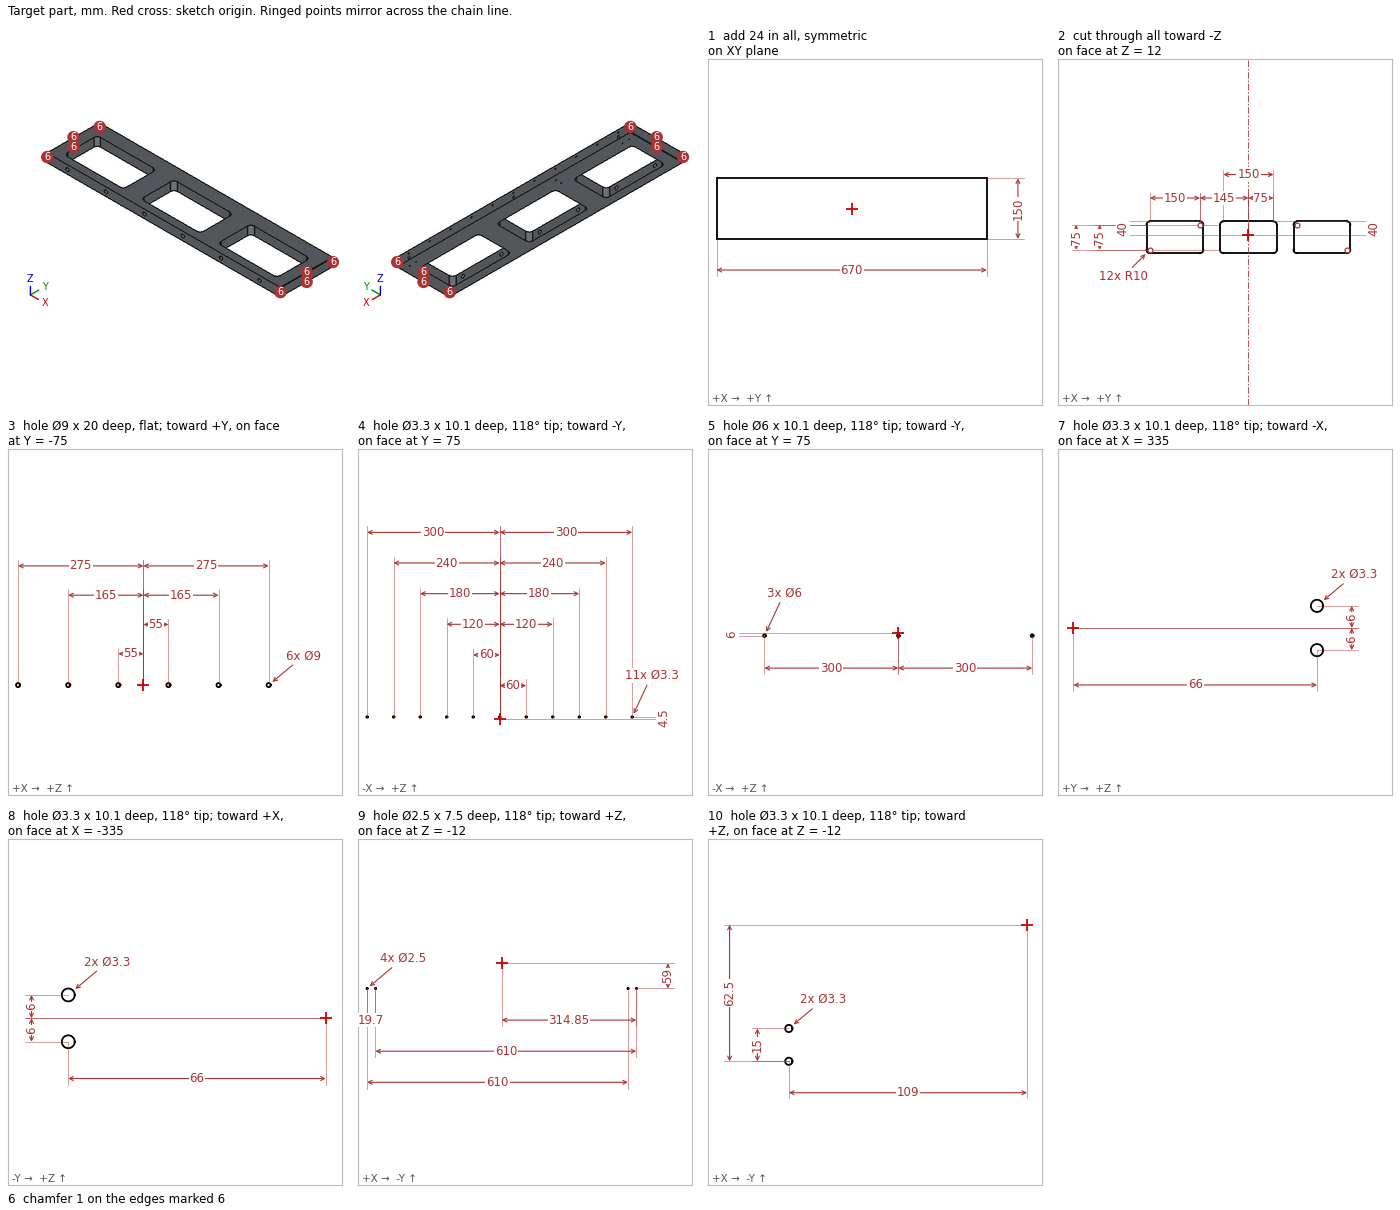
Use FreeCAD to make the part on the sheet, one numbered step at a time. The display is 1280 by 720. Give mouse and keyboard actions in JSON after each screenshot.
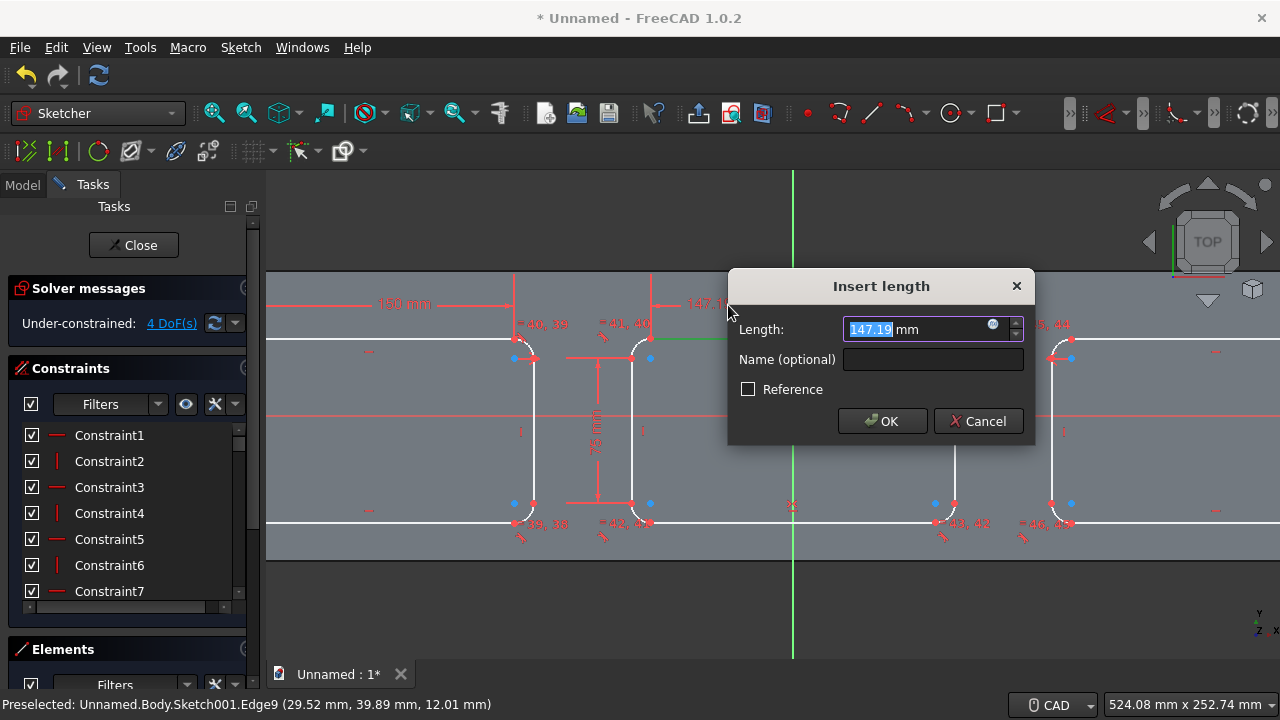
{"action": "type", "text": "150"}
{"action": "key", "text": "Return"}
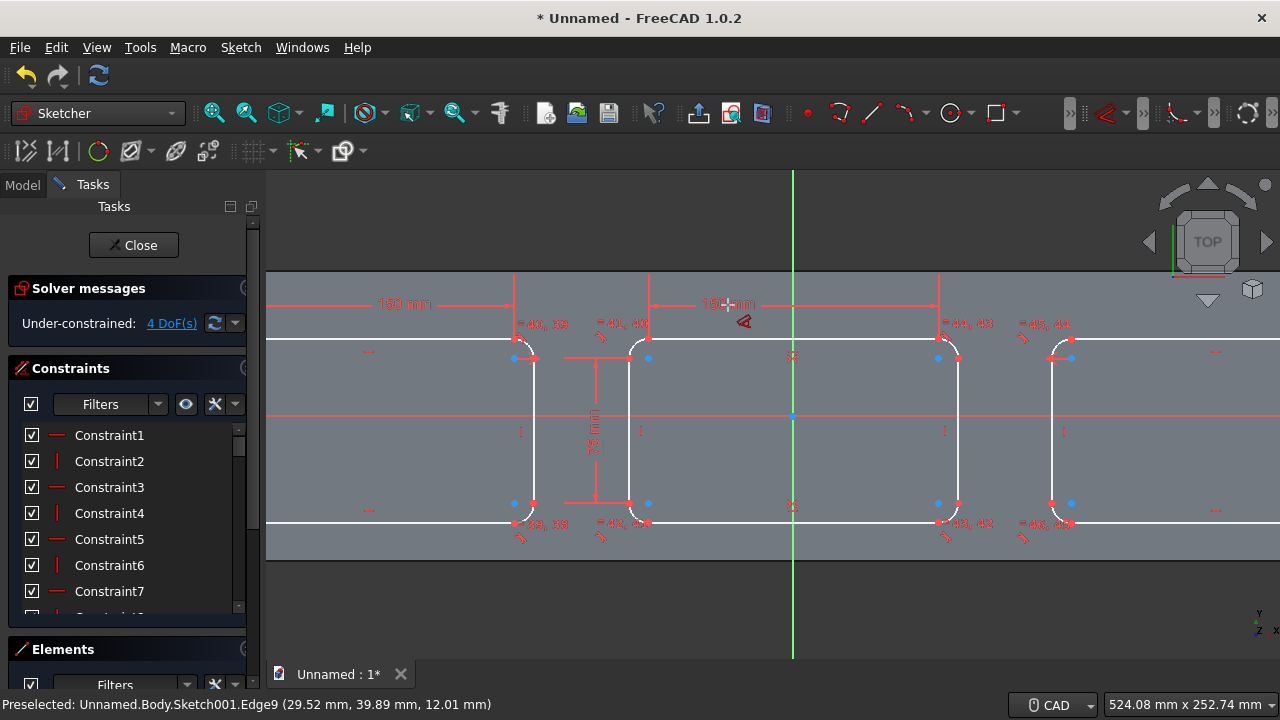
{"action": "left_click", "coordinate": [514, 339]}
{"action": "left_click", "coordinate": [480, 378]}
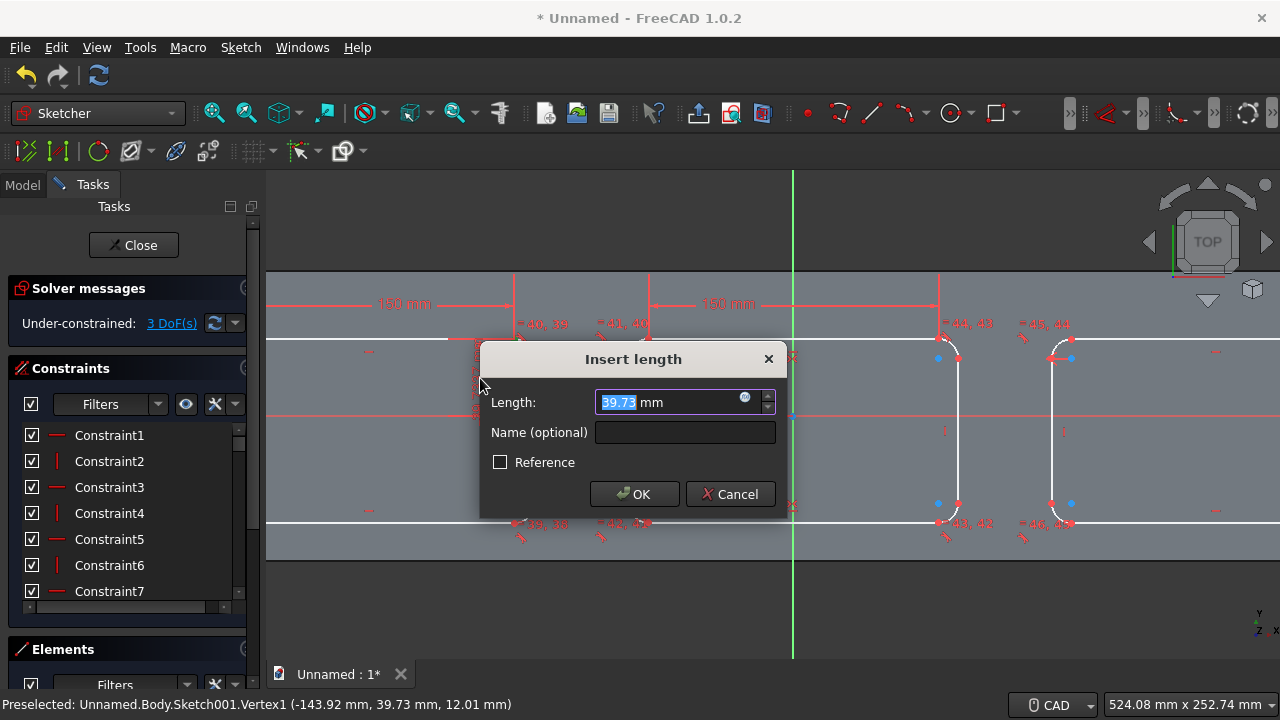
{"action": "type", "text": "40"}
{"action": "key", "text": "Return"}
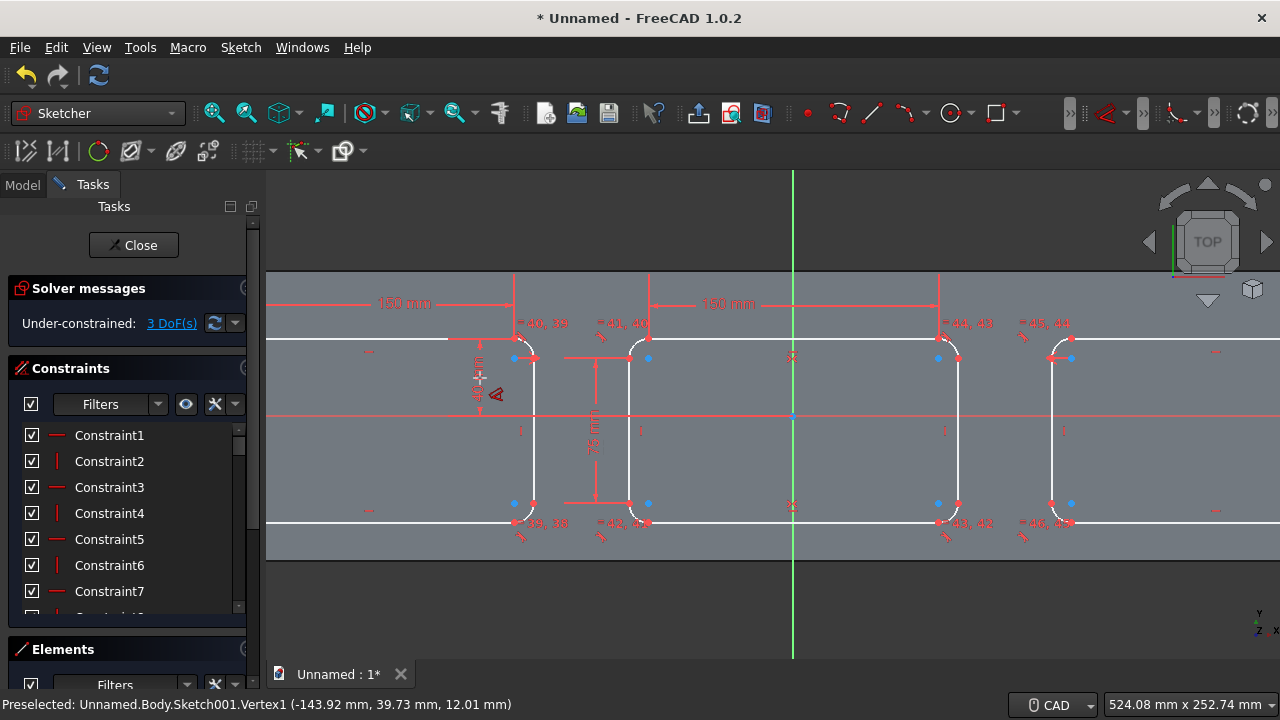
{"action": "left_click", "coordinate": [939, 339]}
{"action": "left_click", "coordinate": [866, 305]}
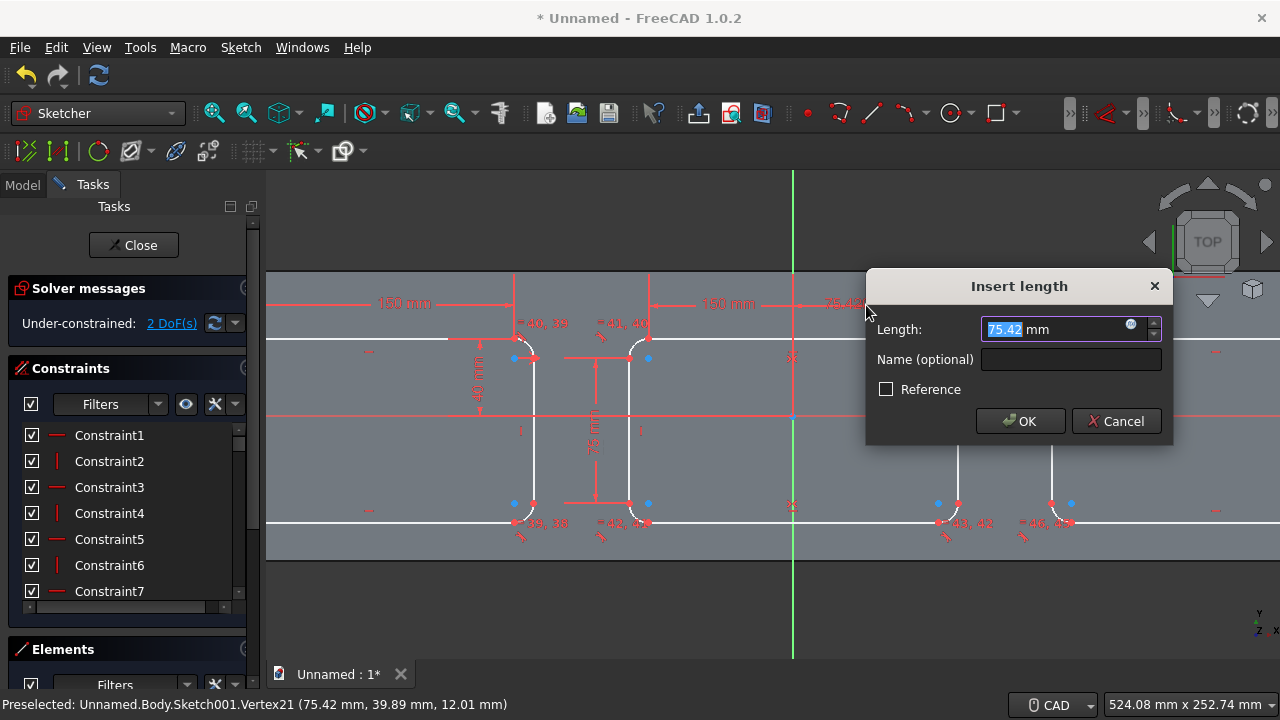
{"action": "type", "text": "75"}
{"action": "key", "text": "Return"}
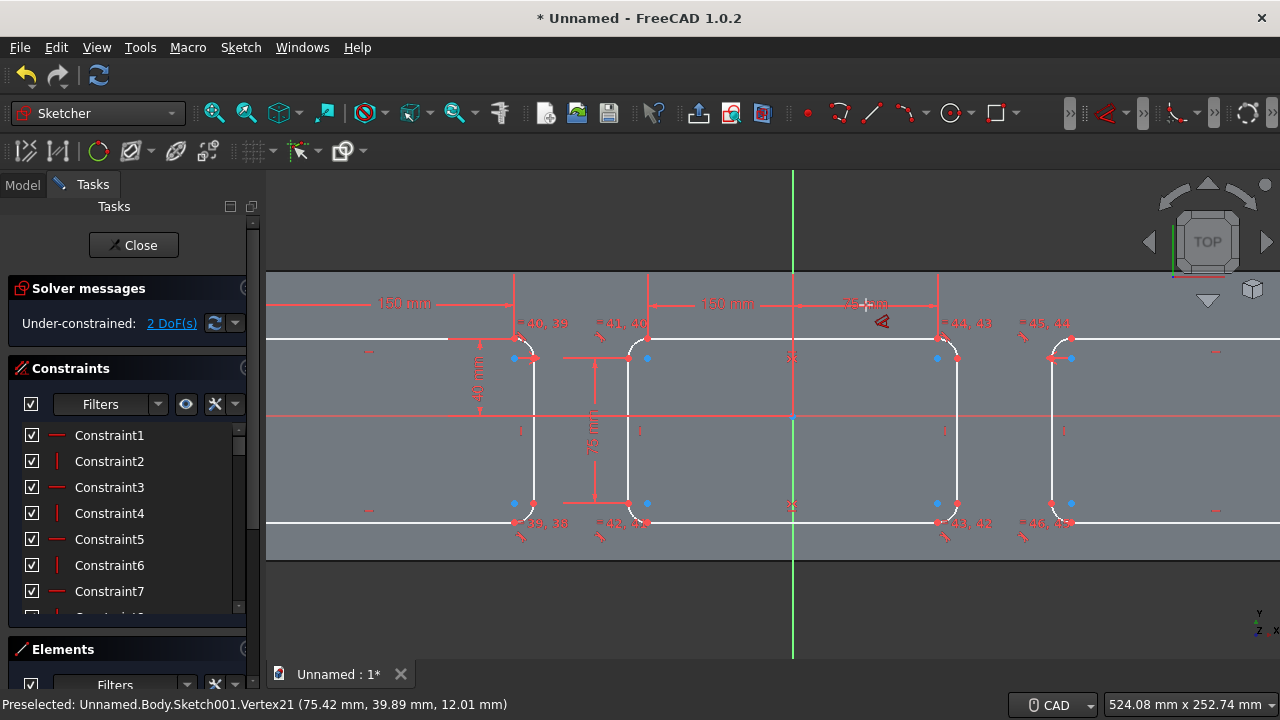
{"action": "left_click", "coordinate": [938, 339]}
{"action": "left_click", "coordinate": [972, 378]}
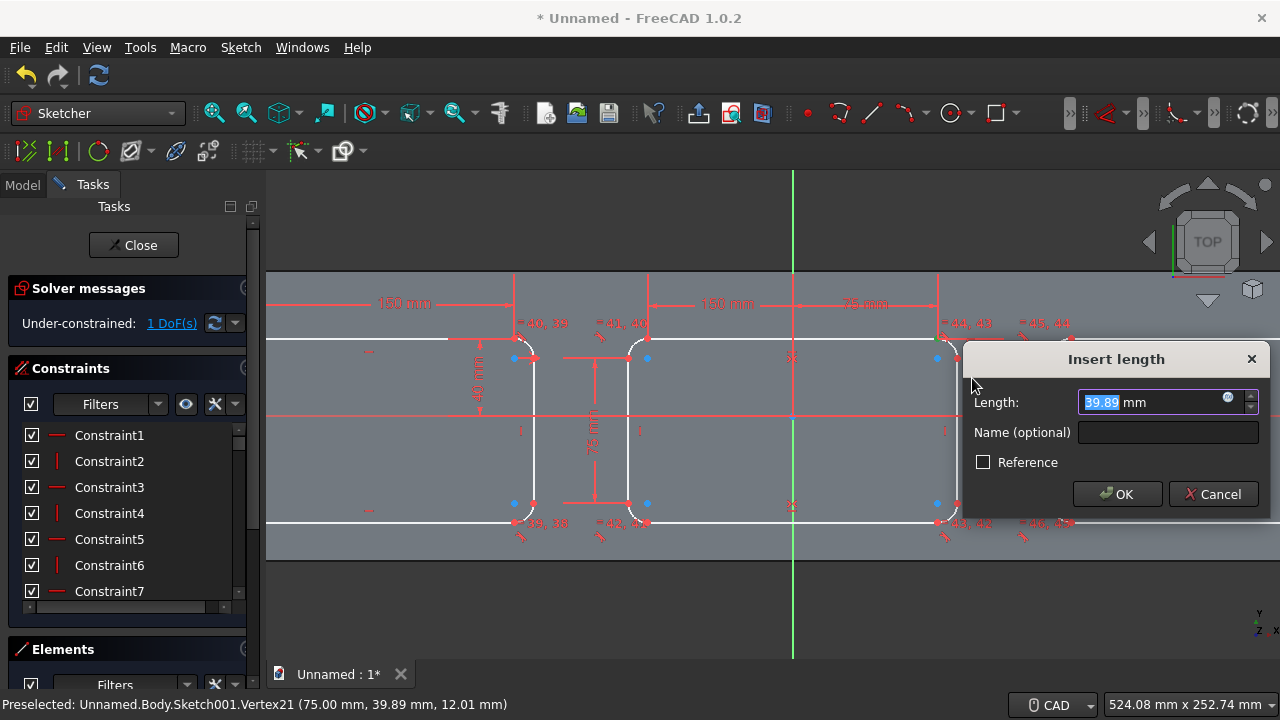
{"action": "type", "text": "40"}
{"action": "key", "text": "Return"}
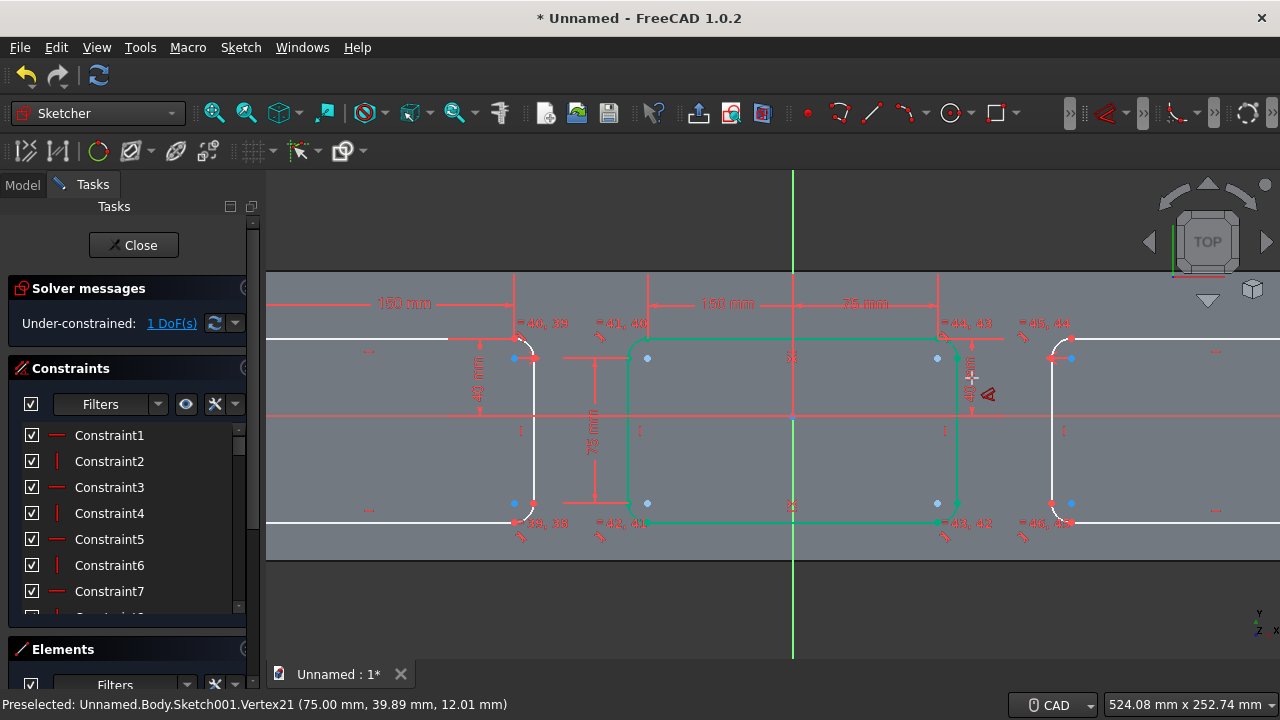
{"action": "left_click", "coordinate": [514, 339]}
{"action": "left_click", "coordinate": [654, 305]}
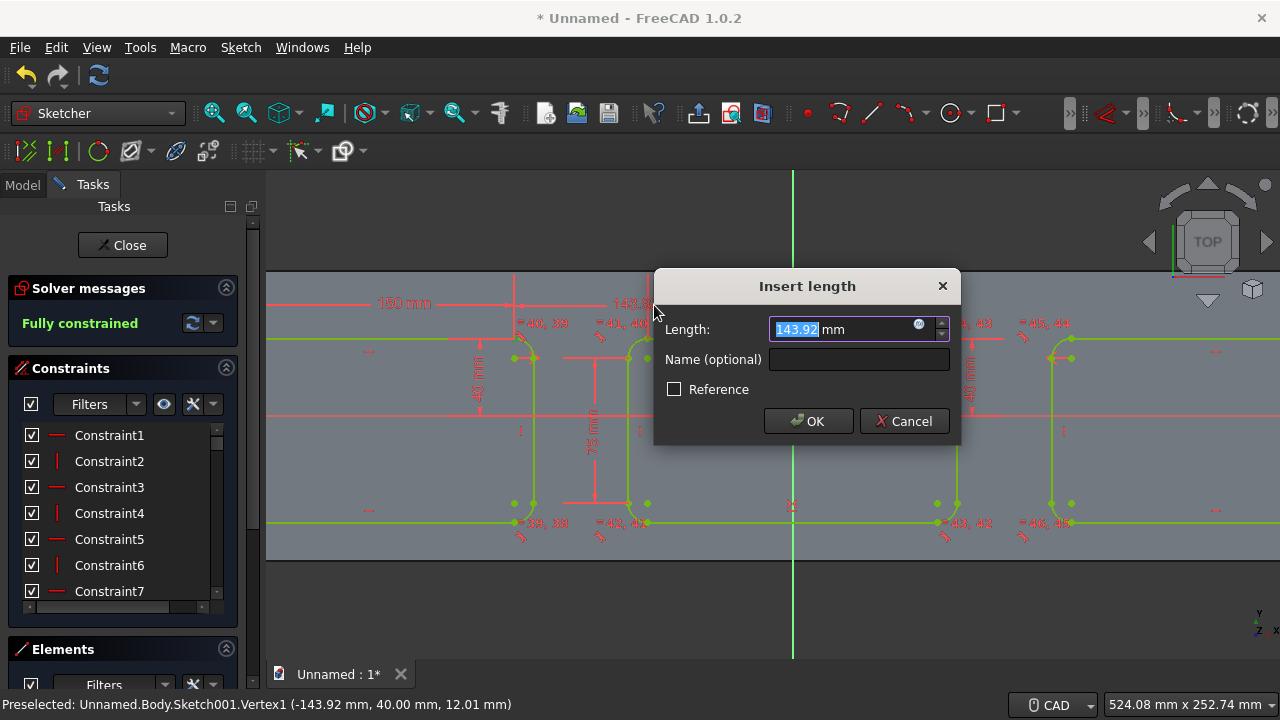
{"action": "type", "text": "145"}
{"action": "key", "text": "Return"}
{"action": "key", "text": "Escape"}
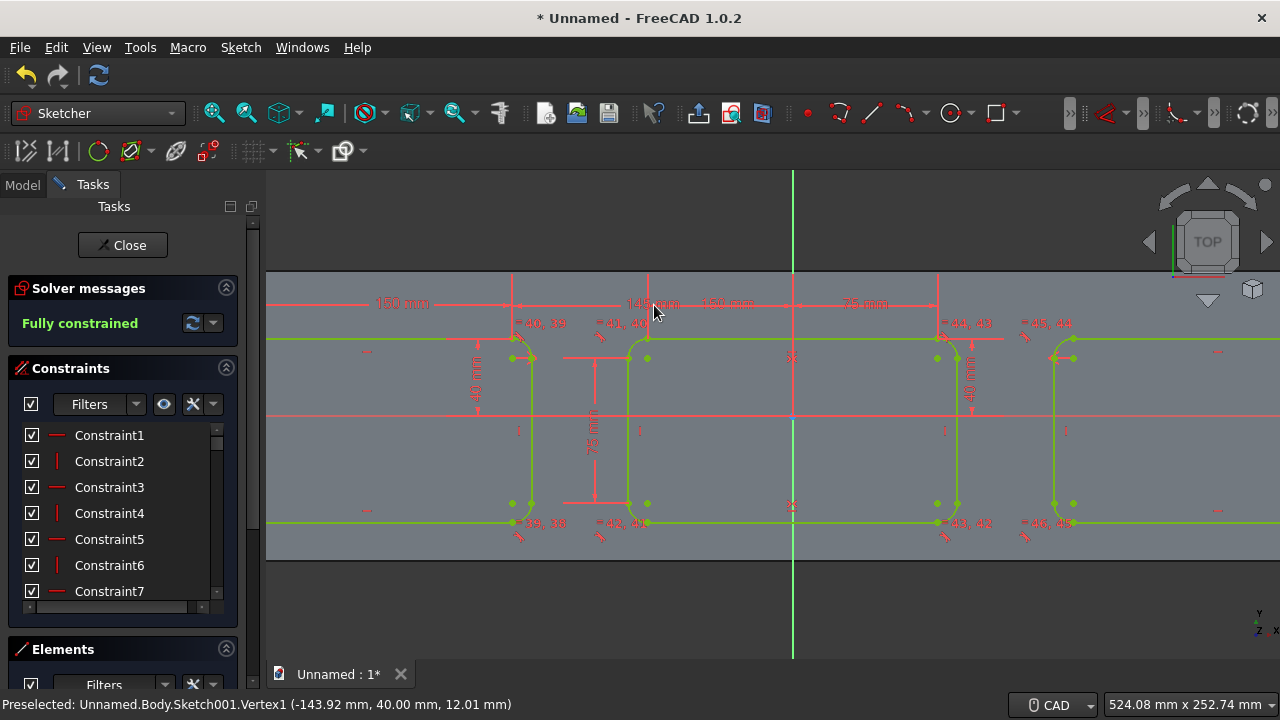
{"action": "left_click", "coordinate": [123, 245]}